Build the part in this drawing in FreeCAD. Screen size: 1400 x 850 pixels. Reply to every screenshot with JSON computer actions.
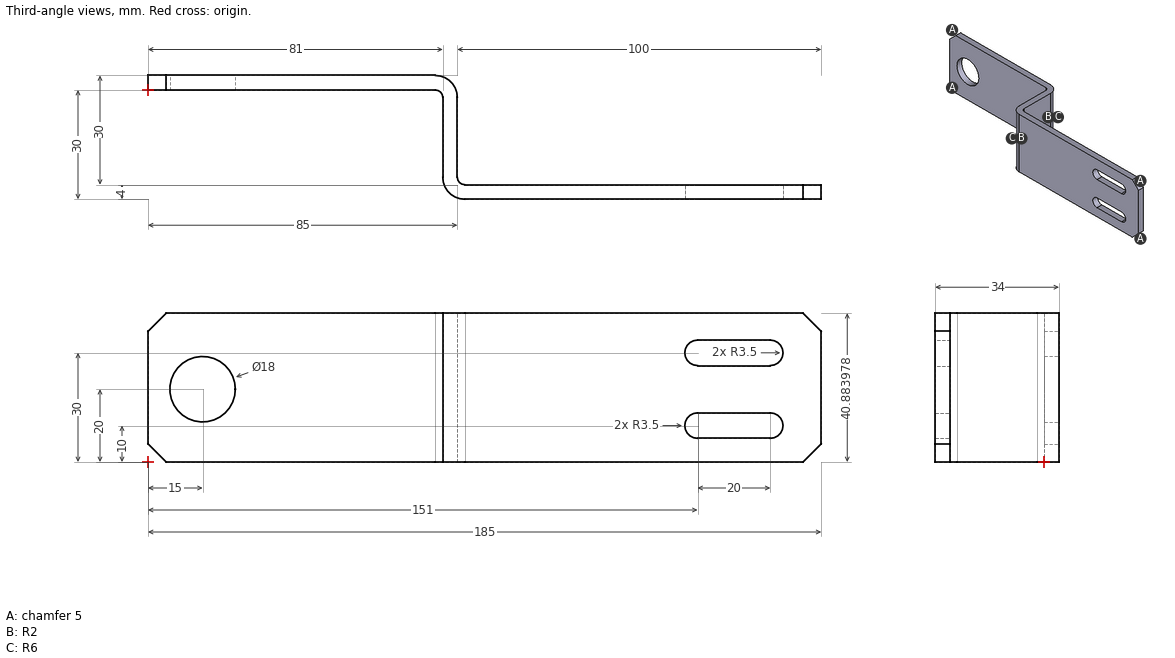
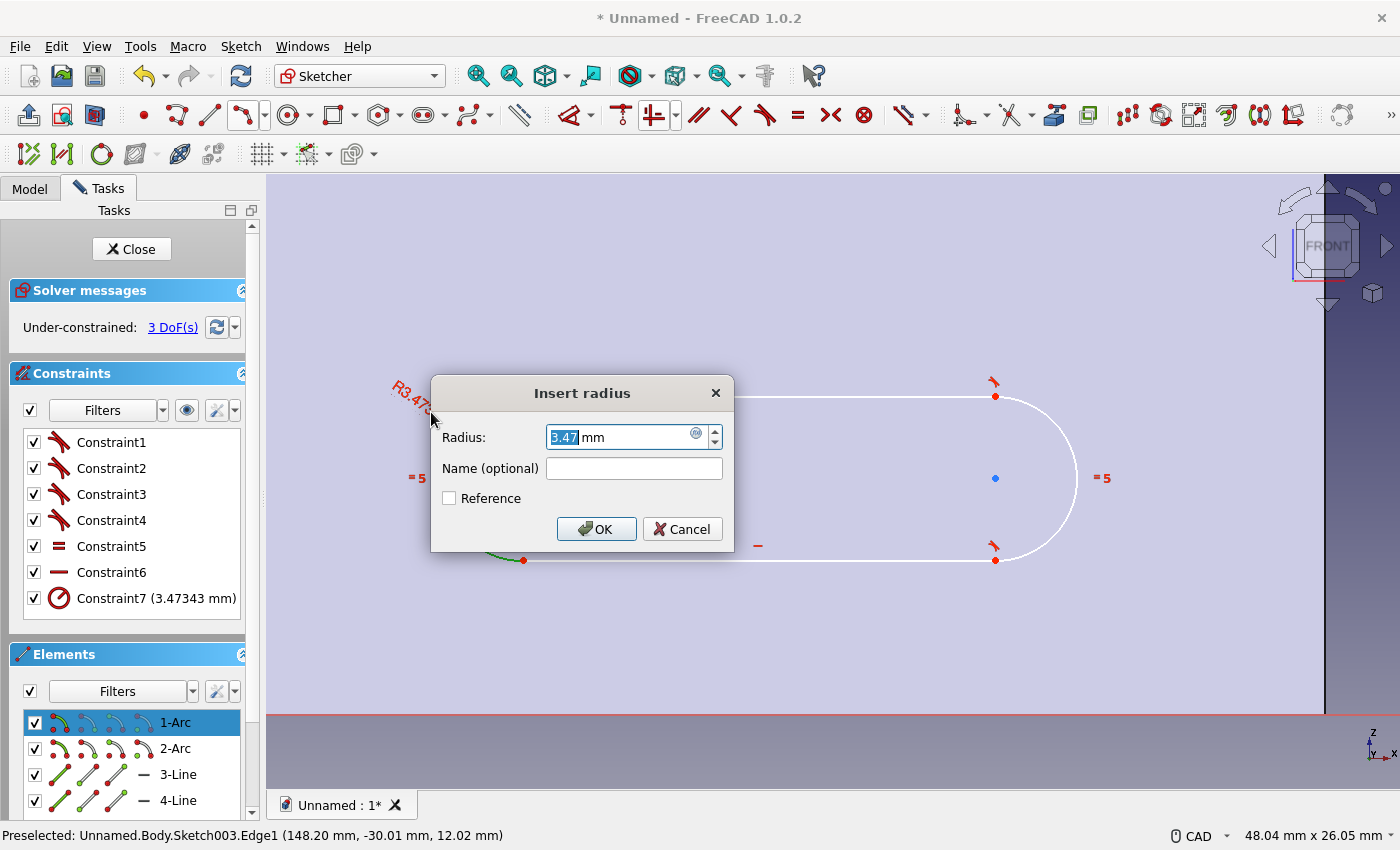
{"action": "type", "text": "3.5"}
{"action": "key", "text": "Return"}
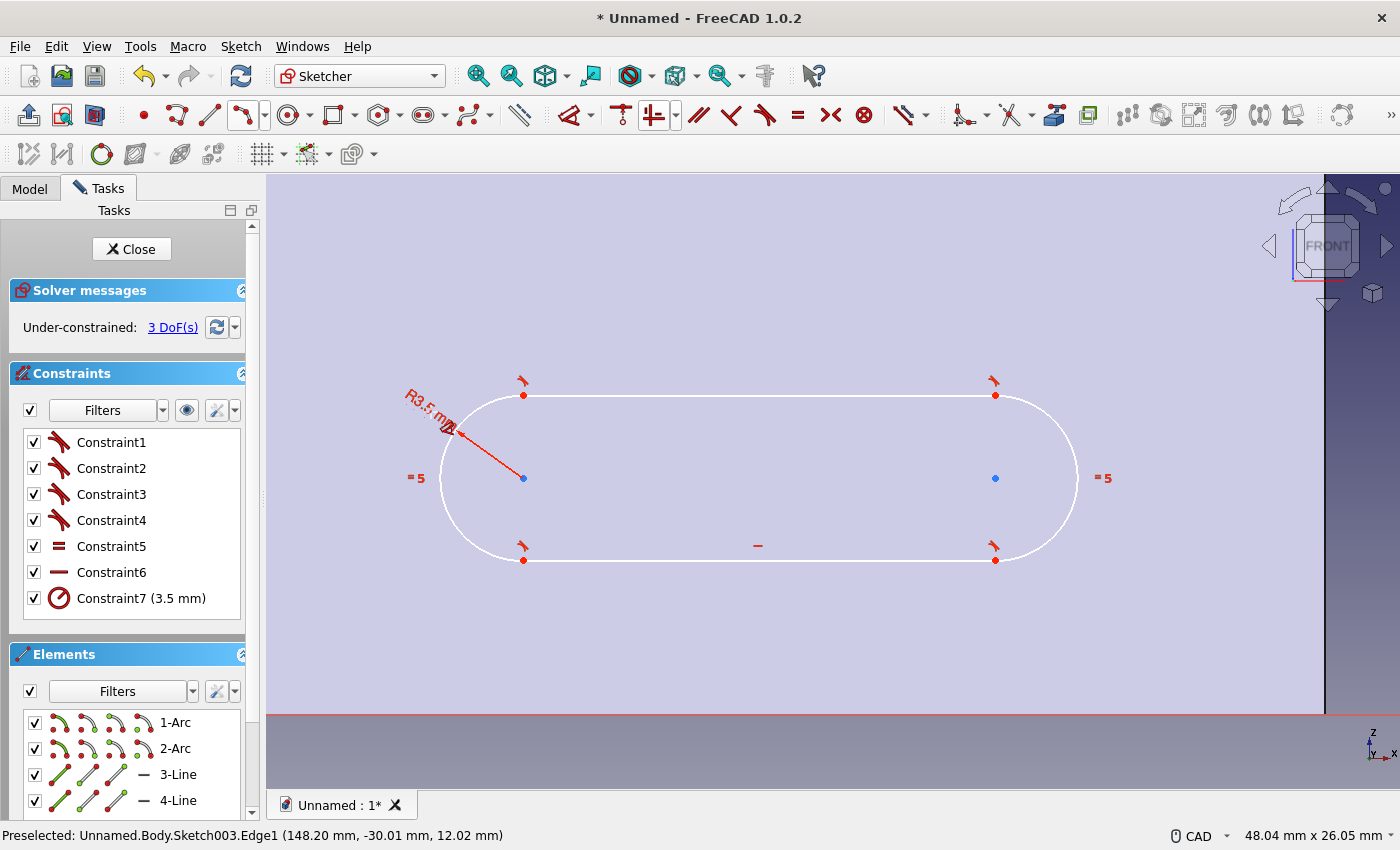
{"action": "left_click", "coordinate": [665, 396]}
{"action": "left_click", "coordinate": [759, 362]}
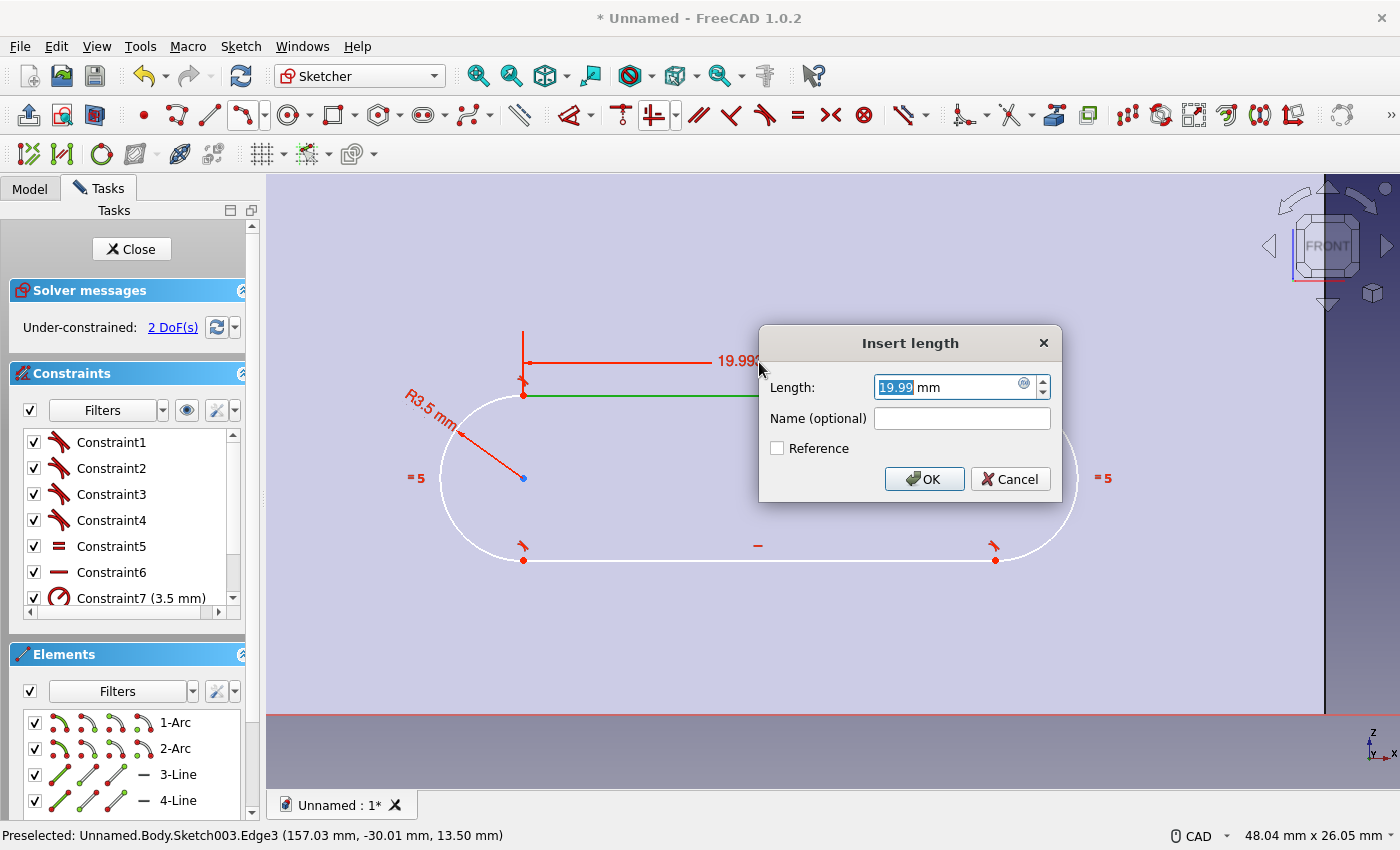
{"action": "type", "text": "20"}
{"action": "key", "text": "Return"}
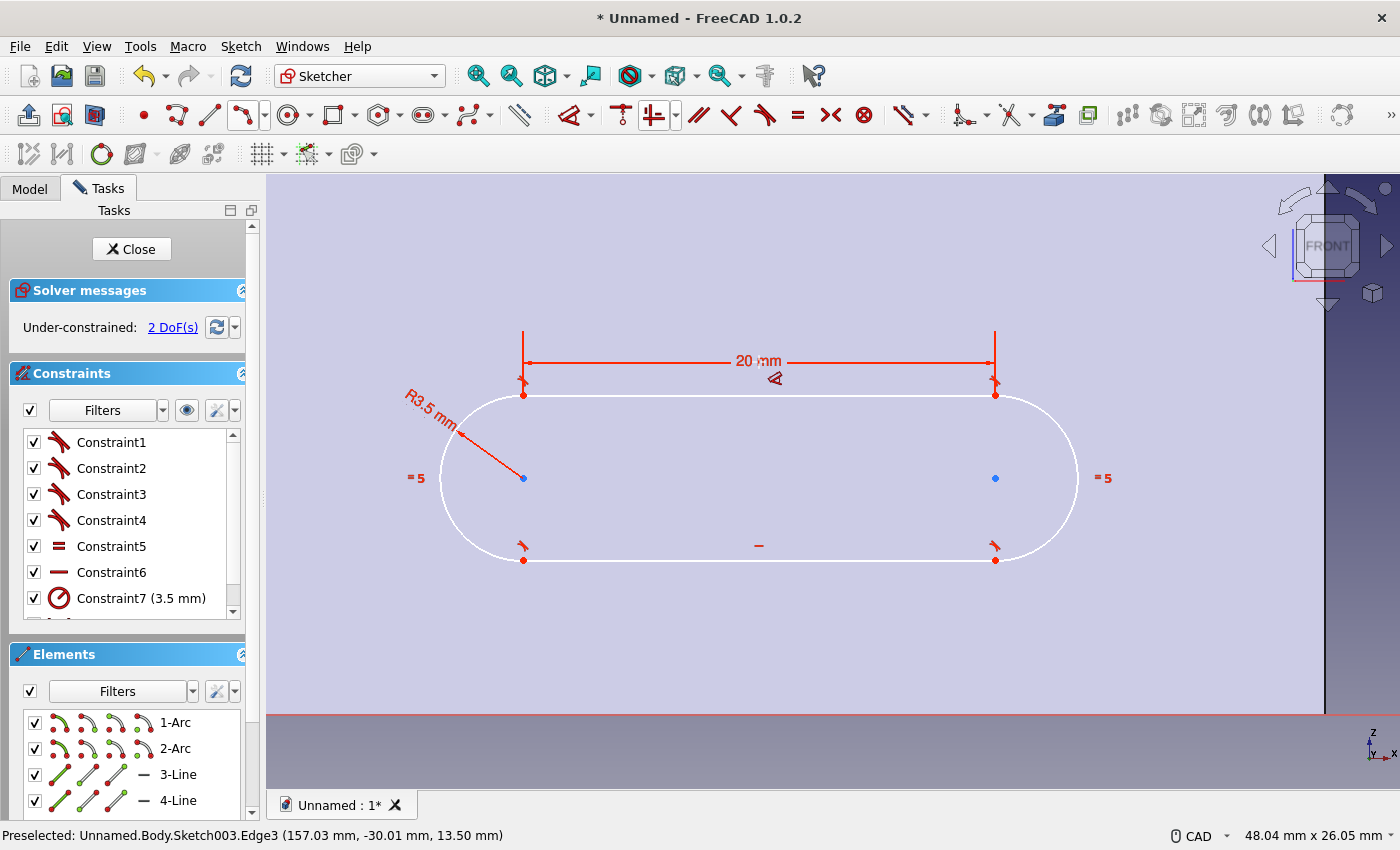
{"action": "left_click", "coordinate": [523, 478]}
{"action": "left_click", "coordinate": [557, 596]}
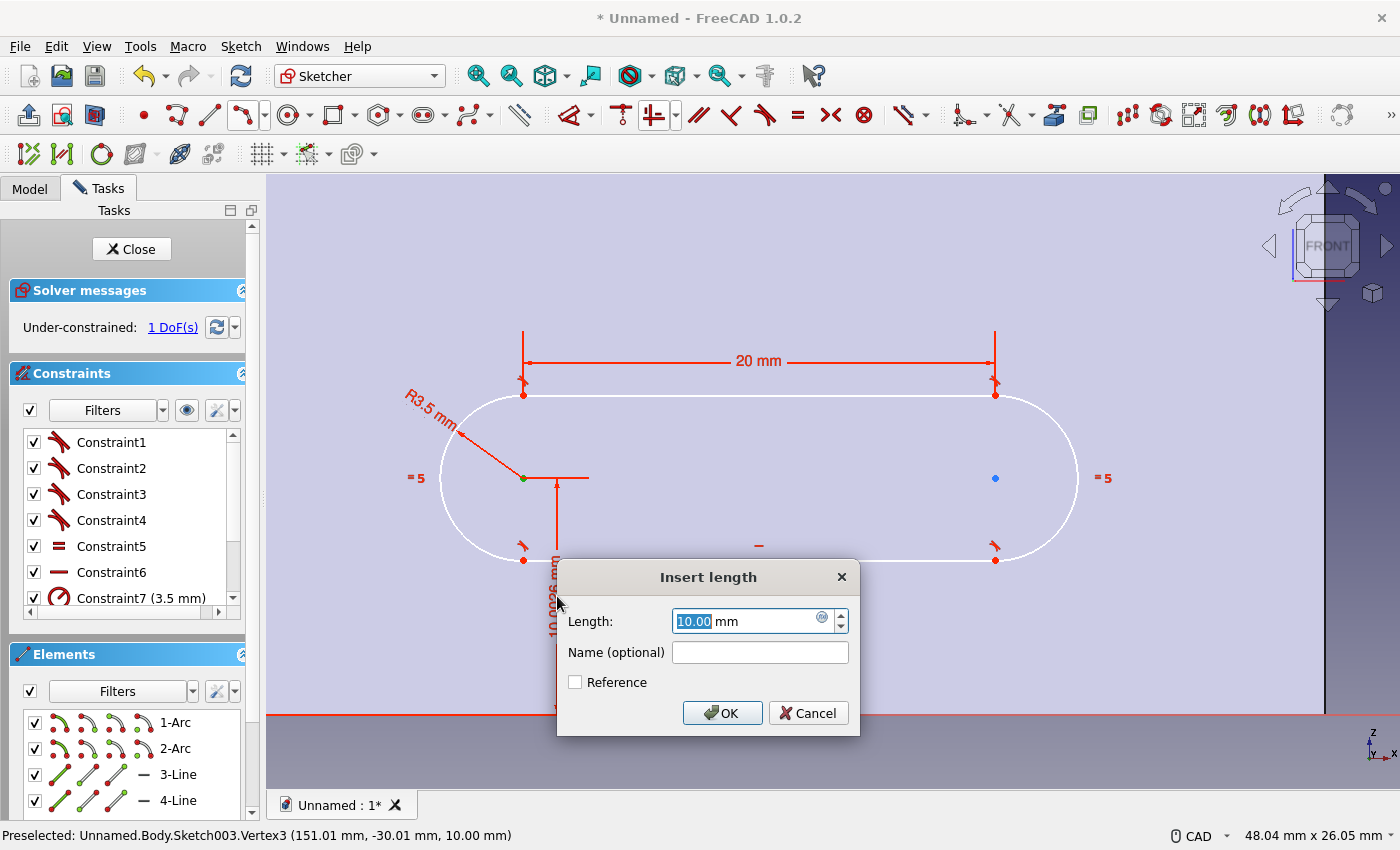
{"action": "type", "text": "10"}
{"action": "key", "text": "Return"}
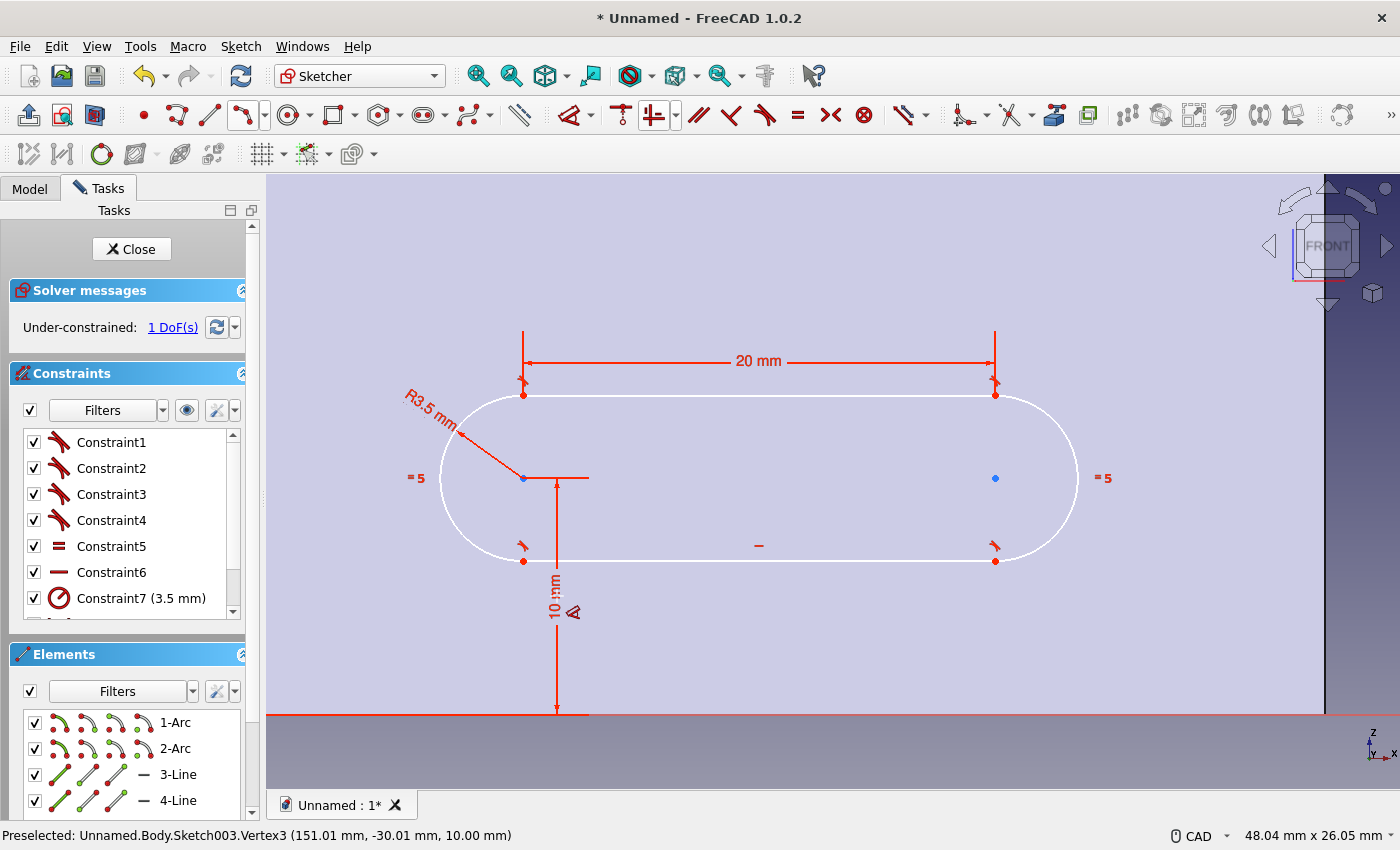
{"action": "left_click", "coordinate": [523, 396]}
{"action": "left_click", "coordinate": [409, 749]}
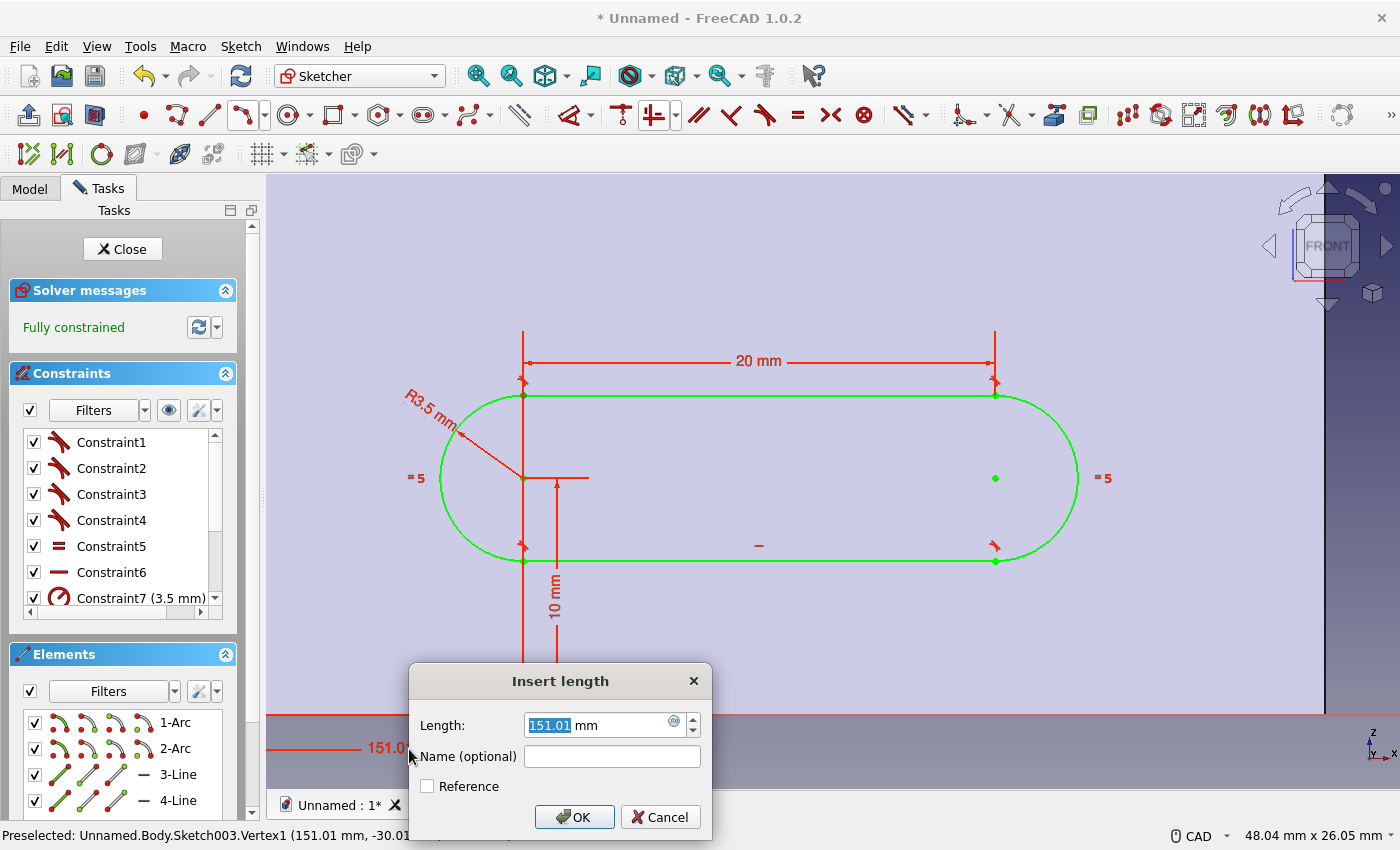
{"action": "type", "text": "151"}
{"action": "key", "text": "Return"}
{"action": "key", "text": "Escape"}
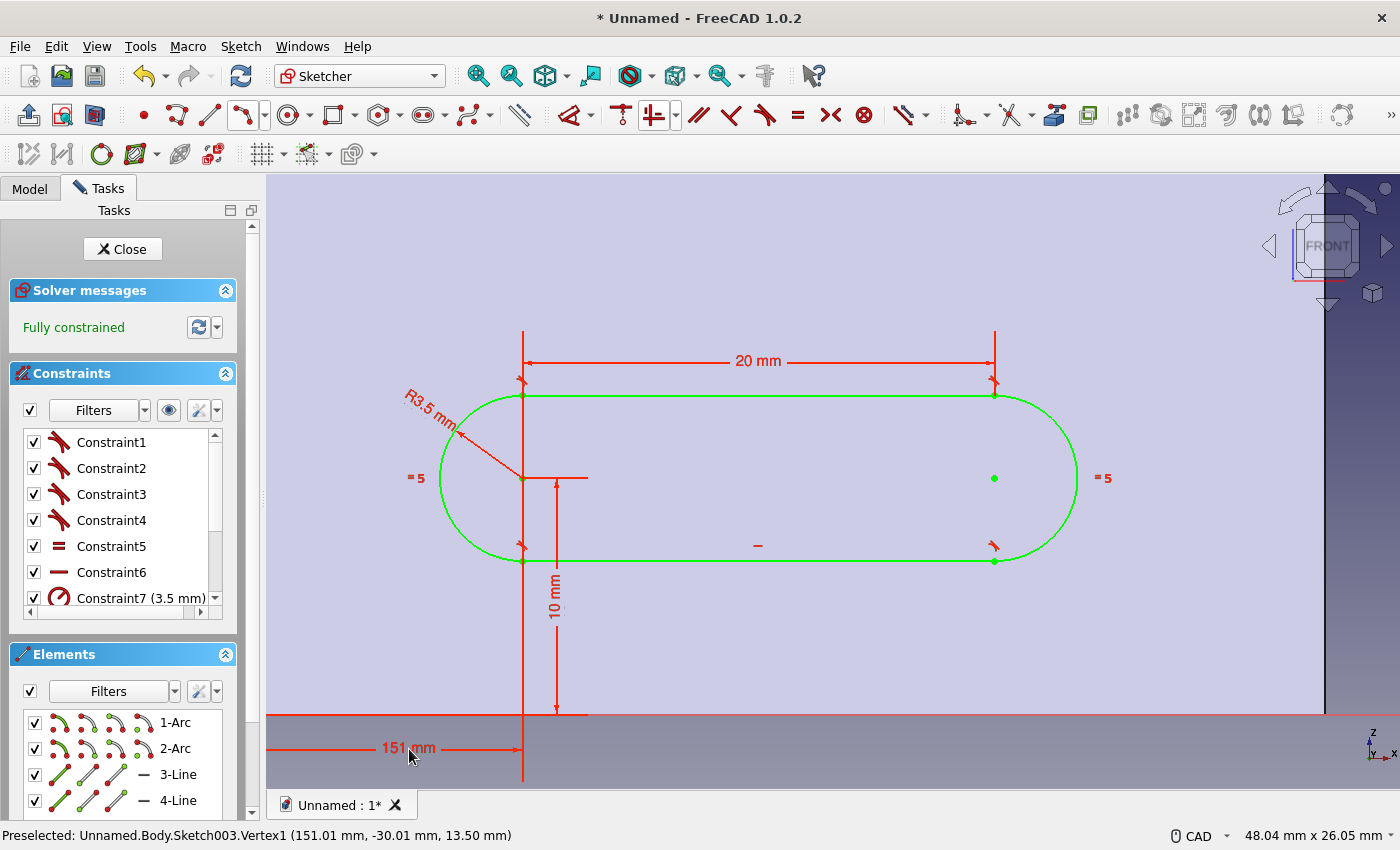
{"action": "left_click", "coordinate": [123, 249]}